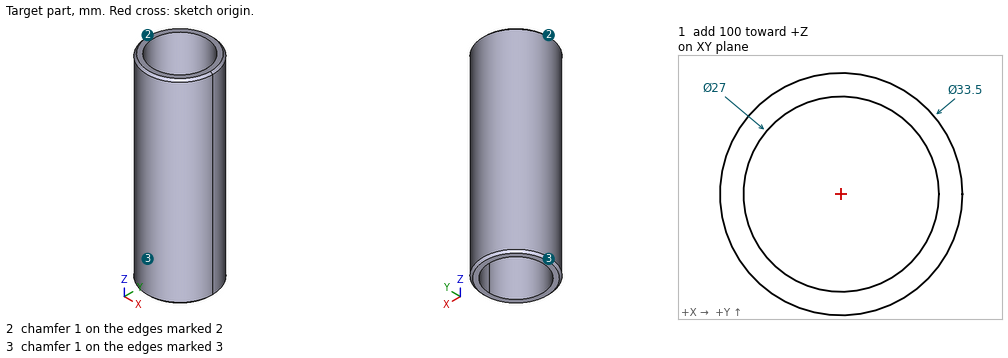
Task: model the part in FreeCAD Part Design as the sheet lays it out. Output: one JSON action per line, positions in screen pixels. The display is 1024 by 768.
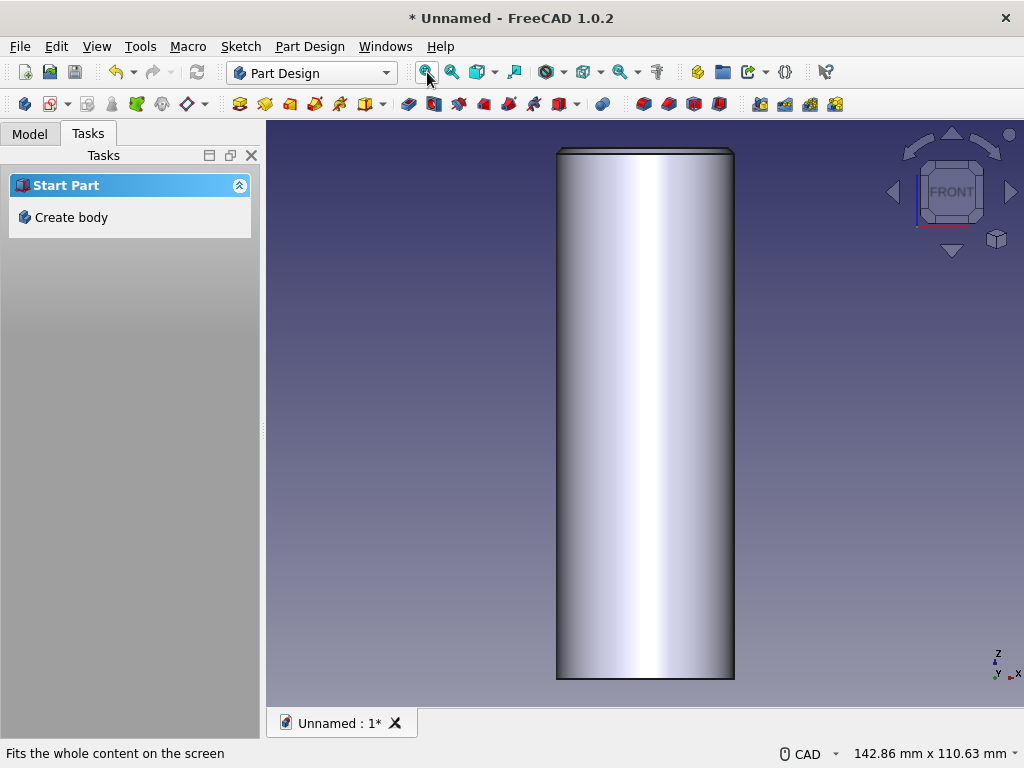
{"action": "left_click", "coordinate": [573, 678]}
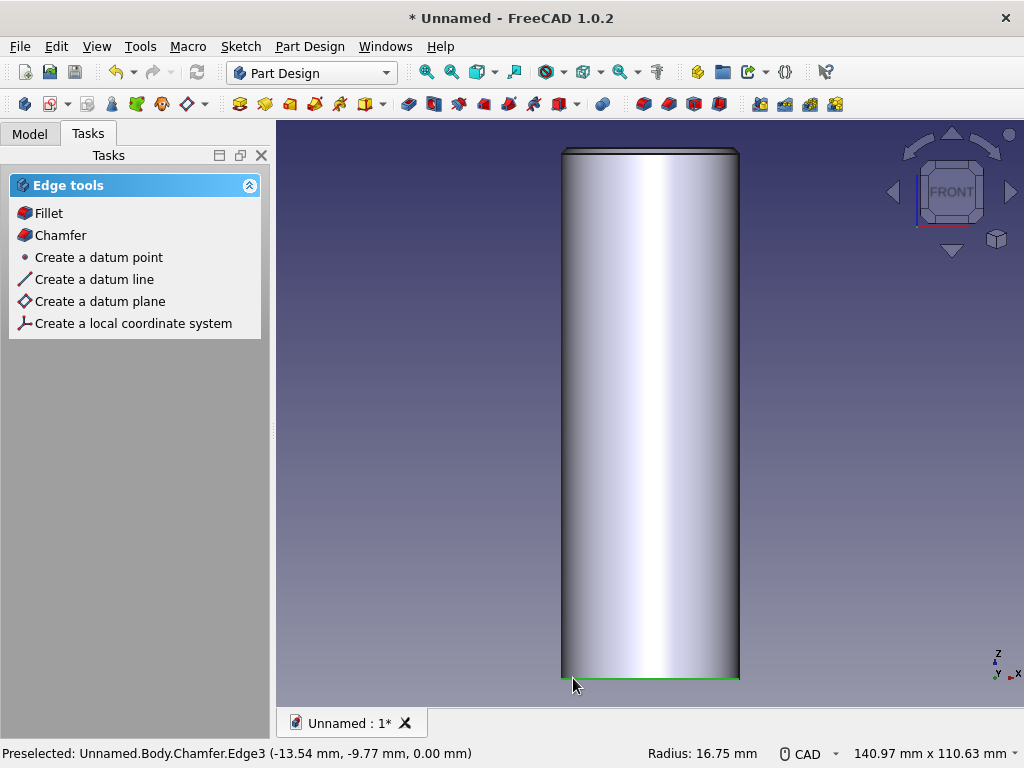
{"action": "left_click", "coordinate": [669, 104]}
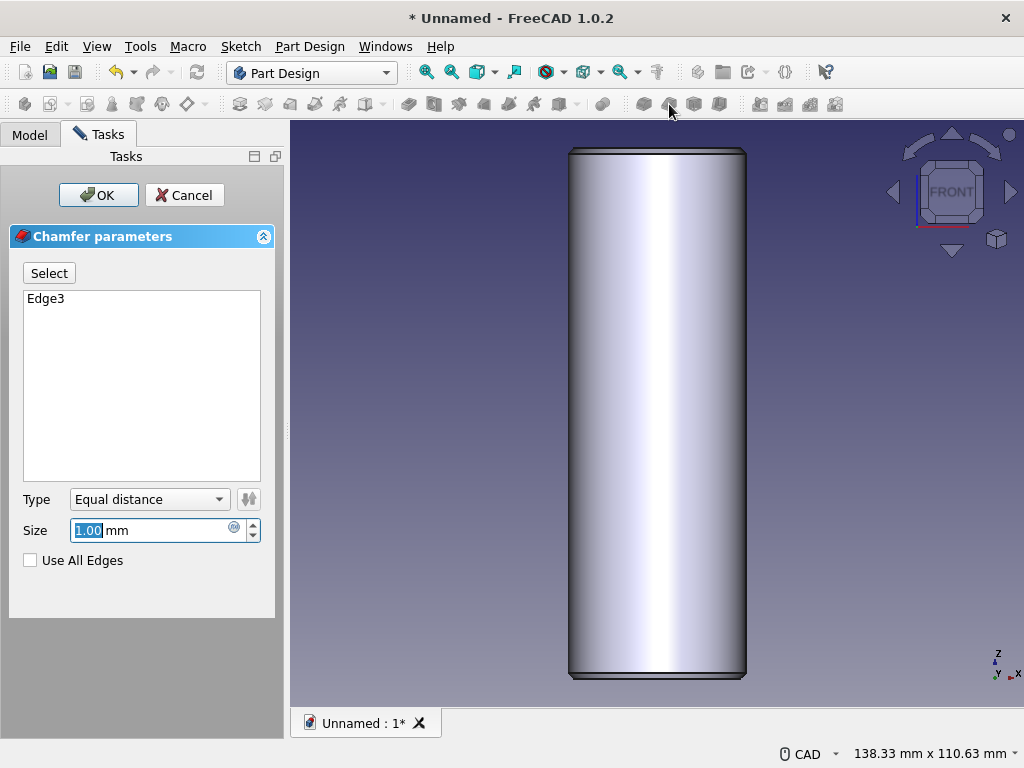
{"action": "type", "text": "1"}
{"action": "key", "text": "Tab"}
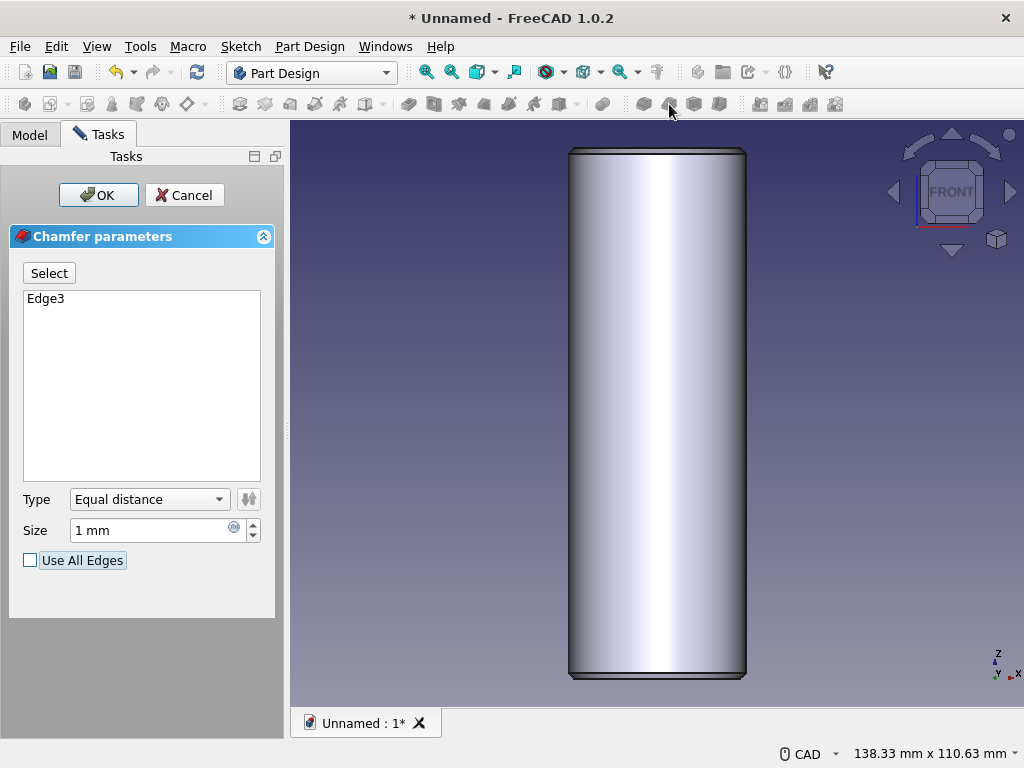
{"action": "left_click", "coordinate": [99, 195]}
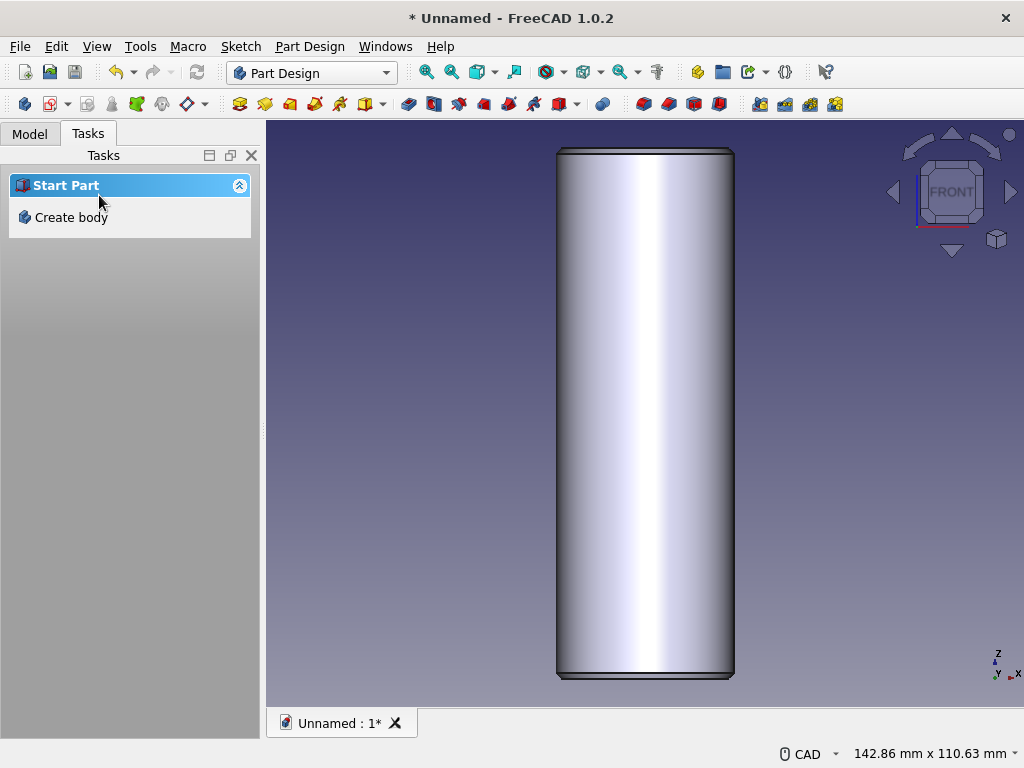
{"action": "key", "text": "0"}